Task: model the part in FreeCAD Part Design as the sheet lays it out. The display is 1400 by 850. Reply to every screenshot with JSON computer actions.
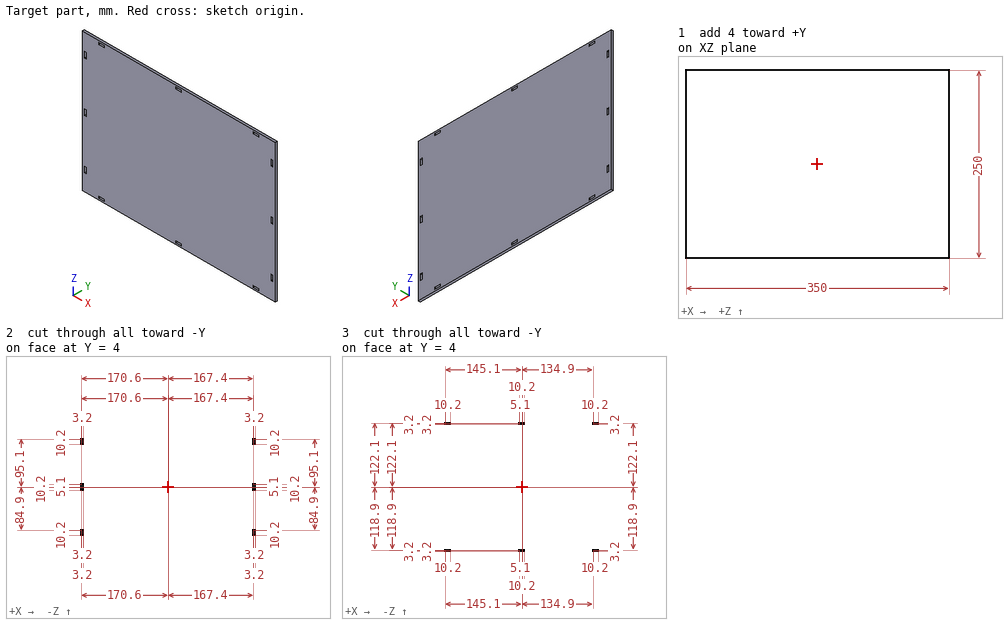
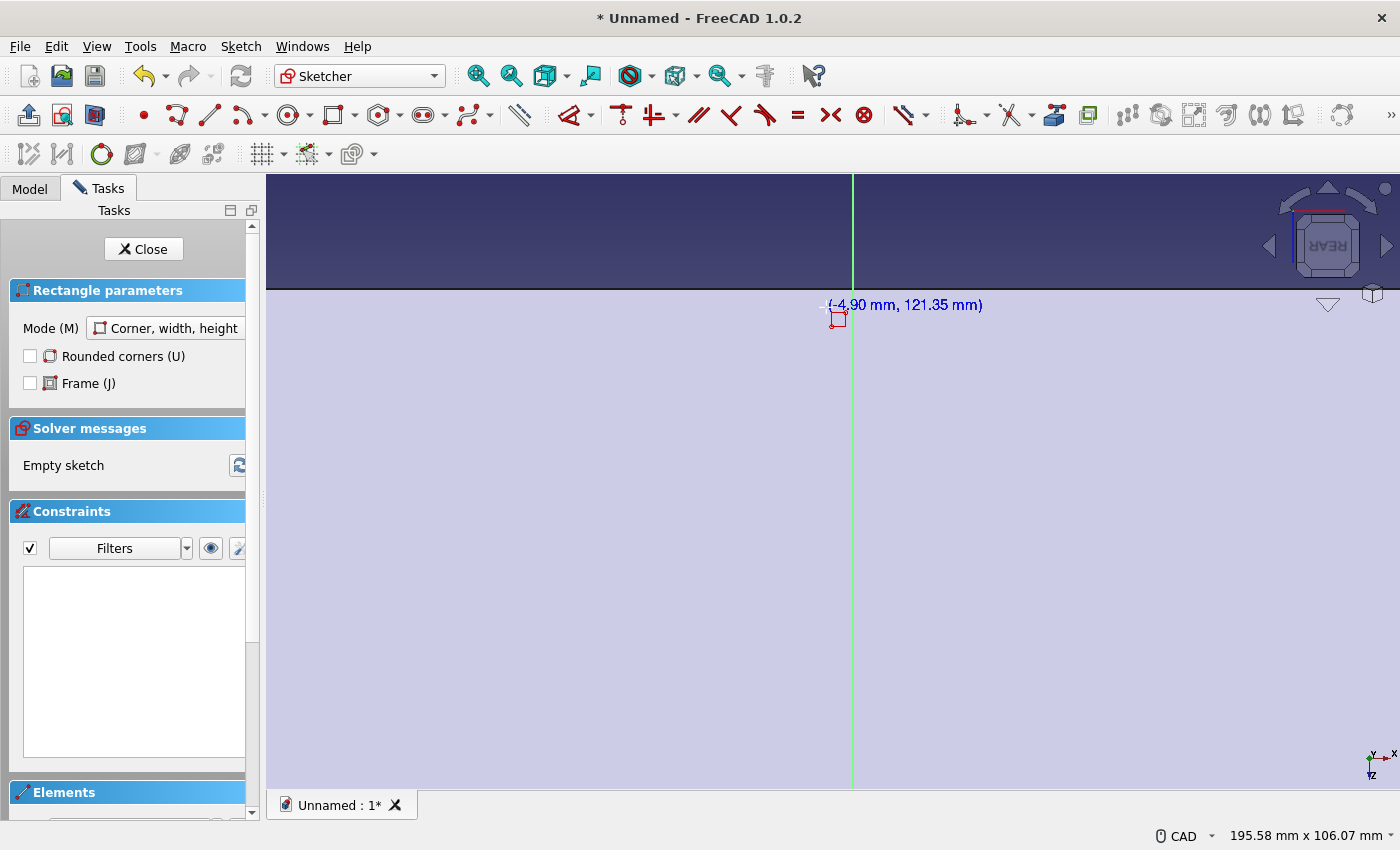
{"action": "left_click", "coordinate": [823, 306]}
{"action": "left_click", "coordinate": [882, 325]}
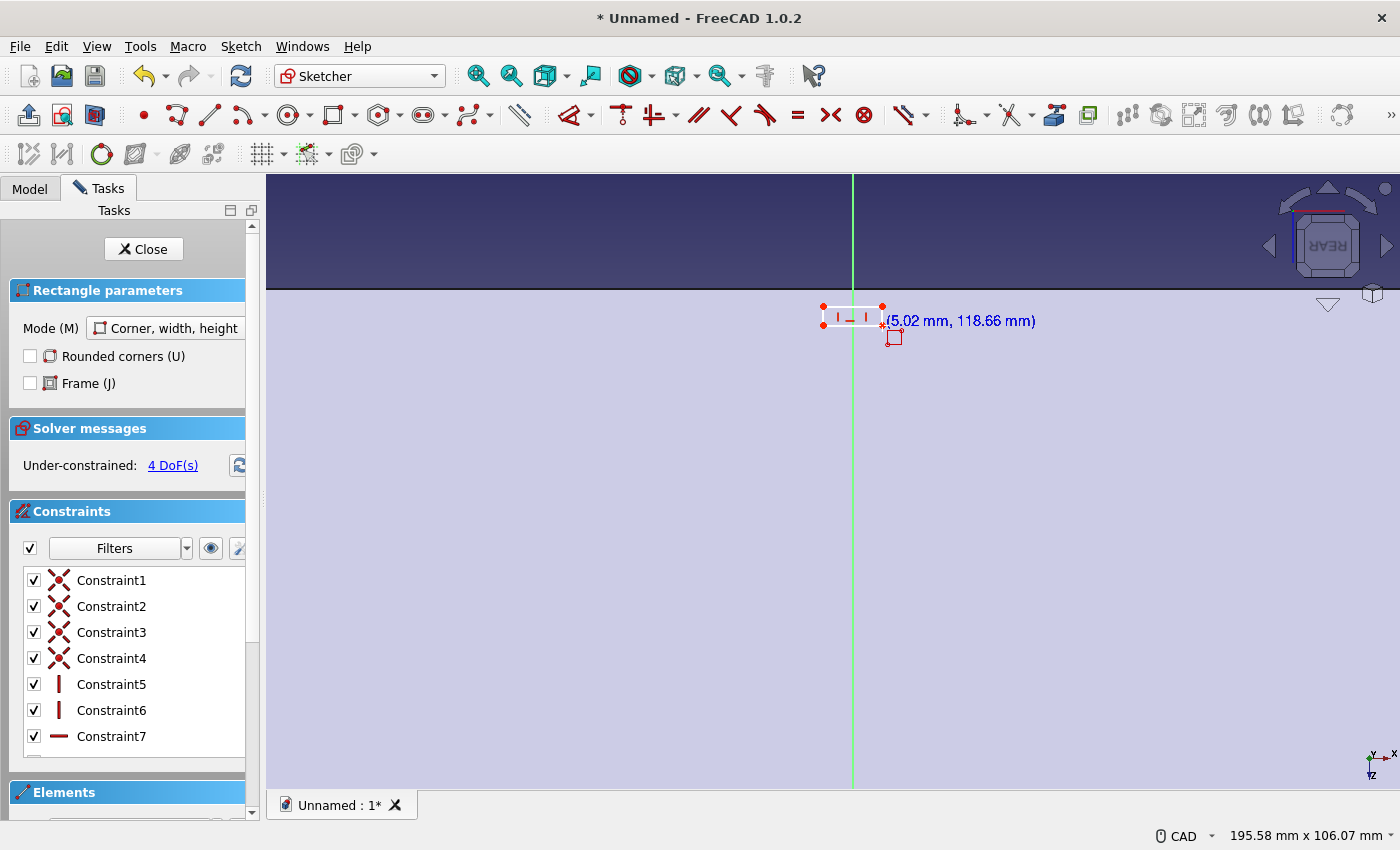
{"action": "scroll", "coordinate": [726, 252], "scroll_direction": "down", "scroll_amount": 6}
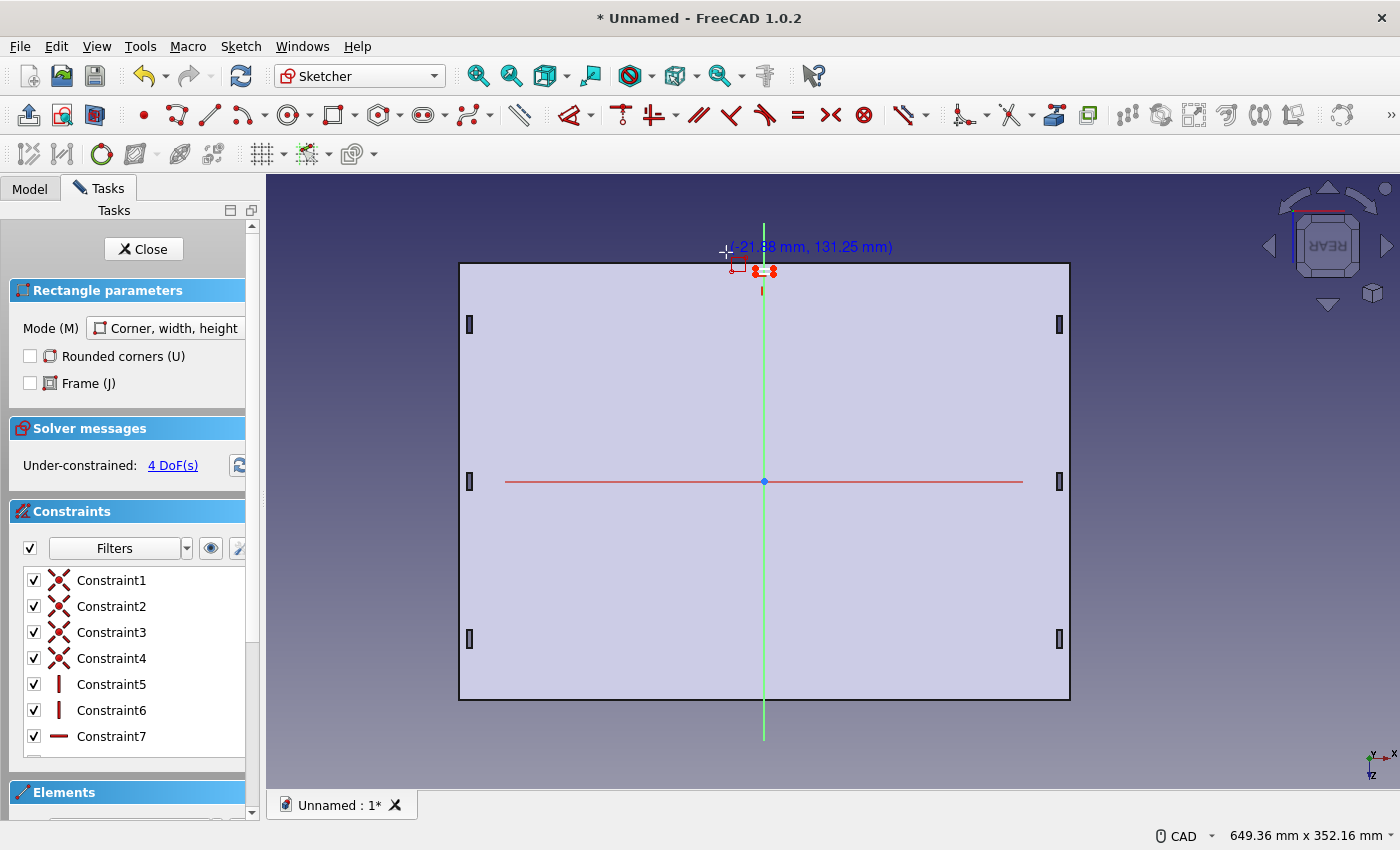
{"action": "scroll", "coordinate": [1000, 268], "scroll_direction": "up", "scroll_amount": 6}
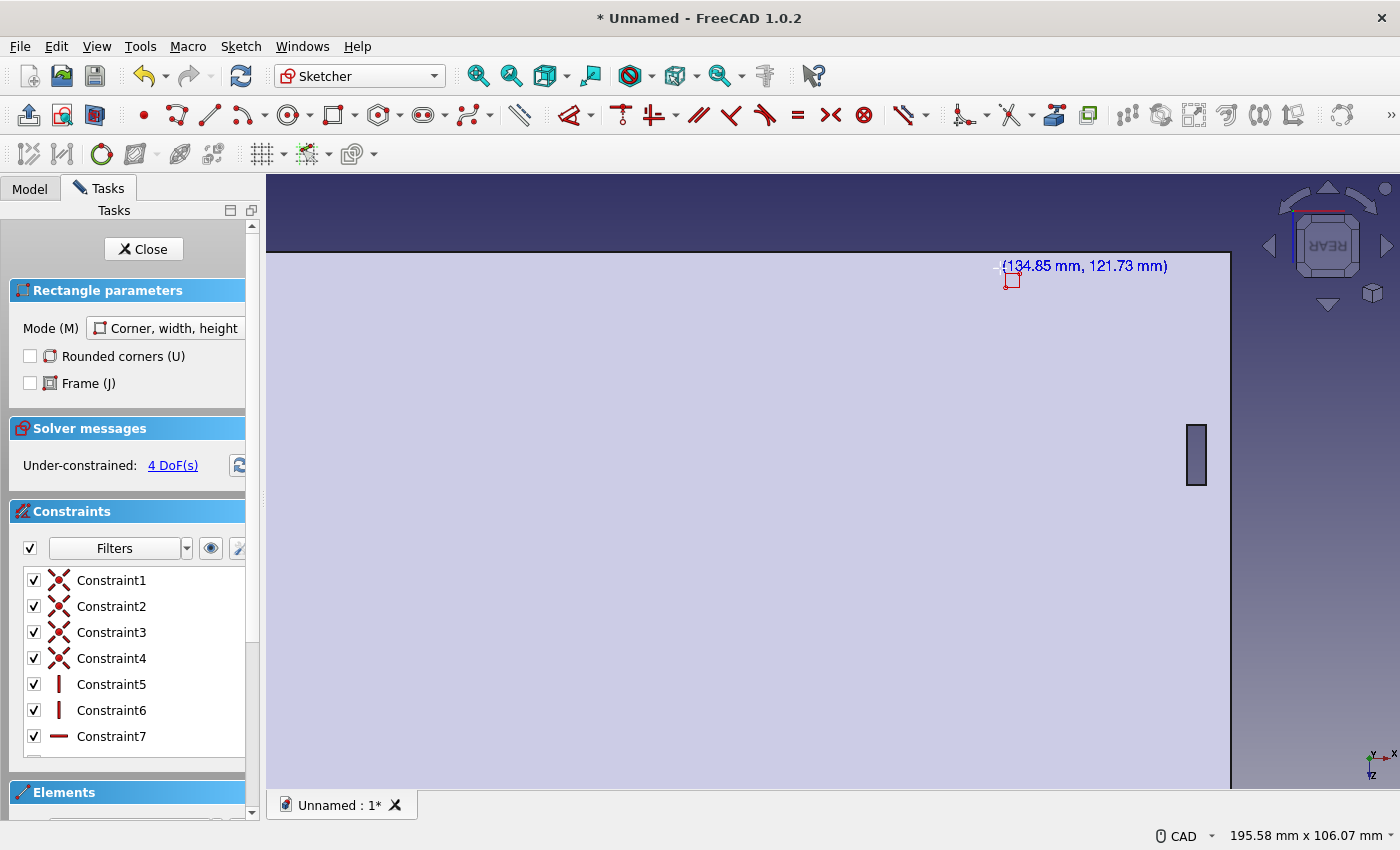
{"action": "scroll", "coordinate": [1001, 268], "scroll_direction": "down", "scroll_amount": 6}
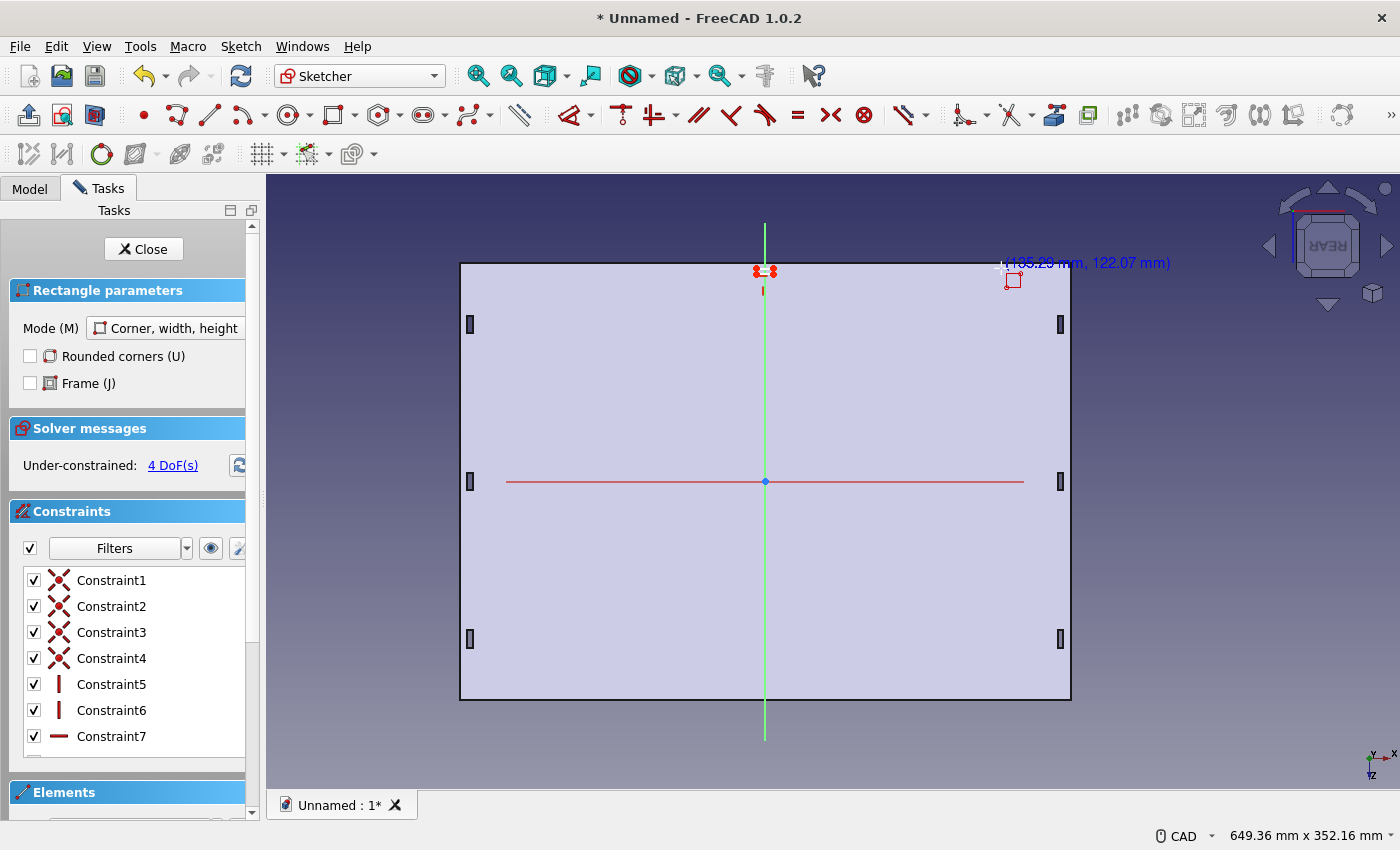
{"action": "left_click", "coordinate": [1001, 268]}
{"action": "left_click", "coordinate": [1019, 274]}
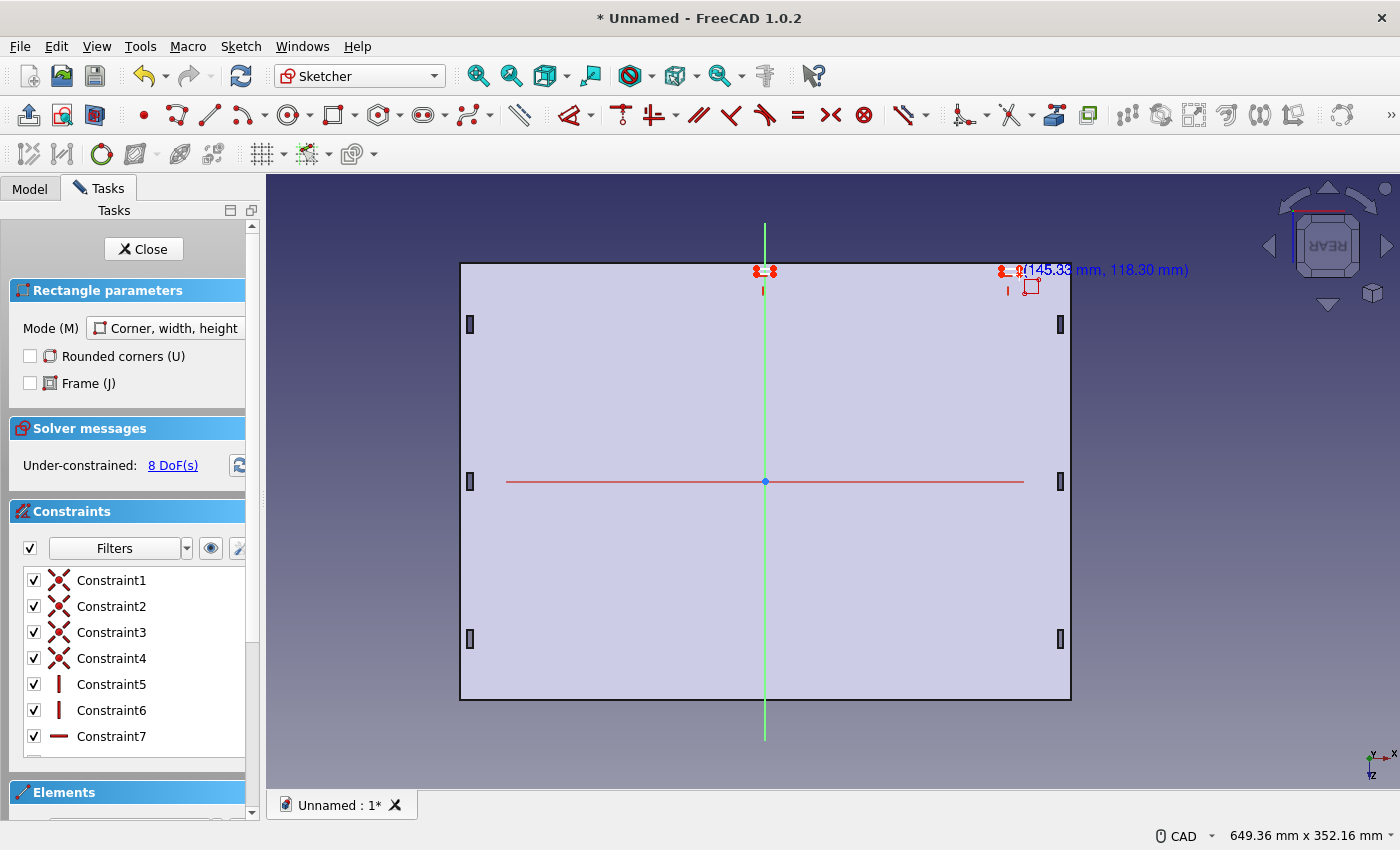
{"action": "scroll", "coordinate": [512, 268], "scroll_direction": "up", "scroll_amount": 6}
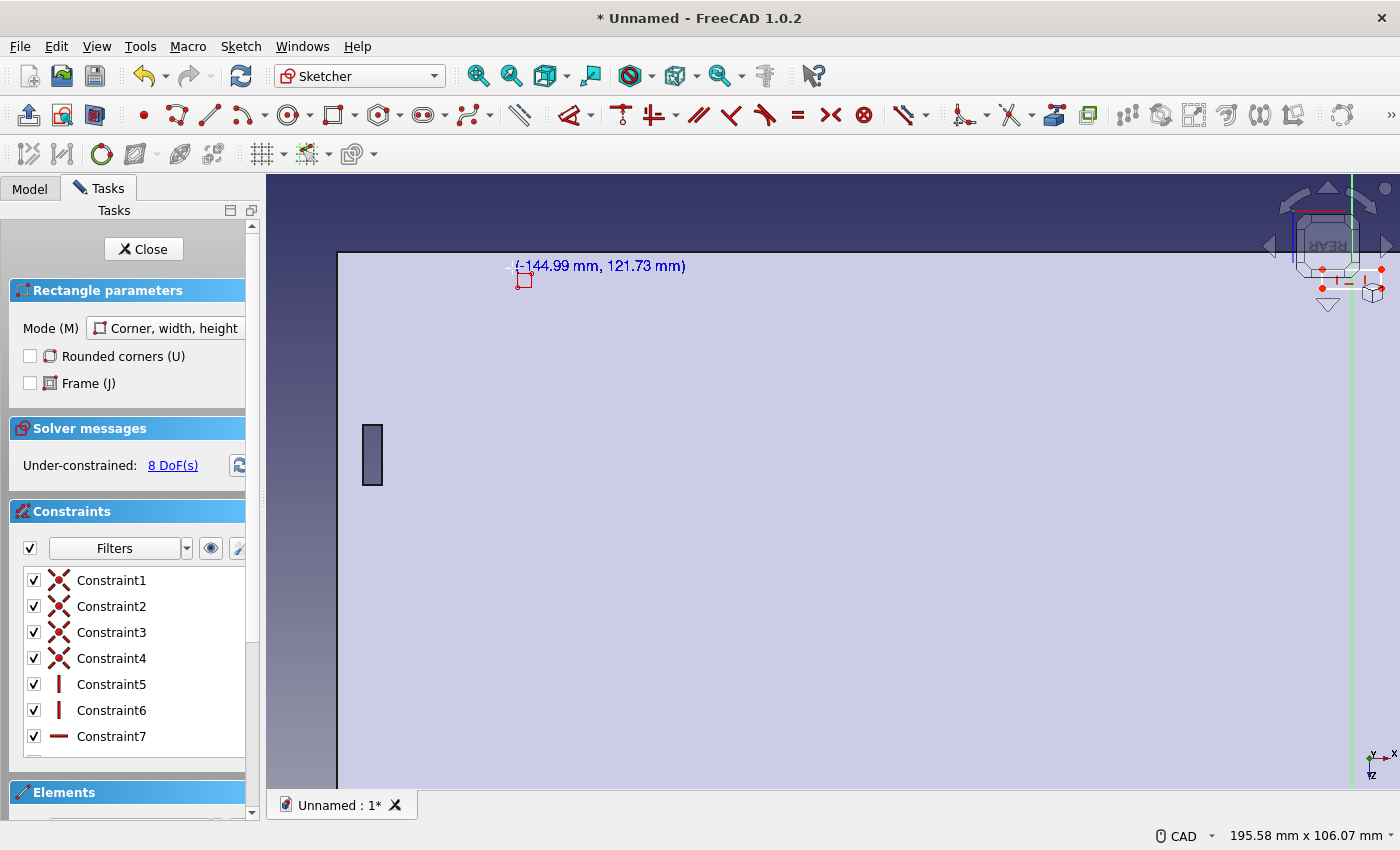
{"action": "scroll", "coordinate": [511, 268], "scroll_direction": "down", "scroll_amount": 6}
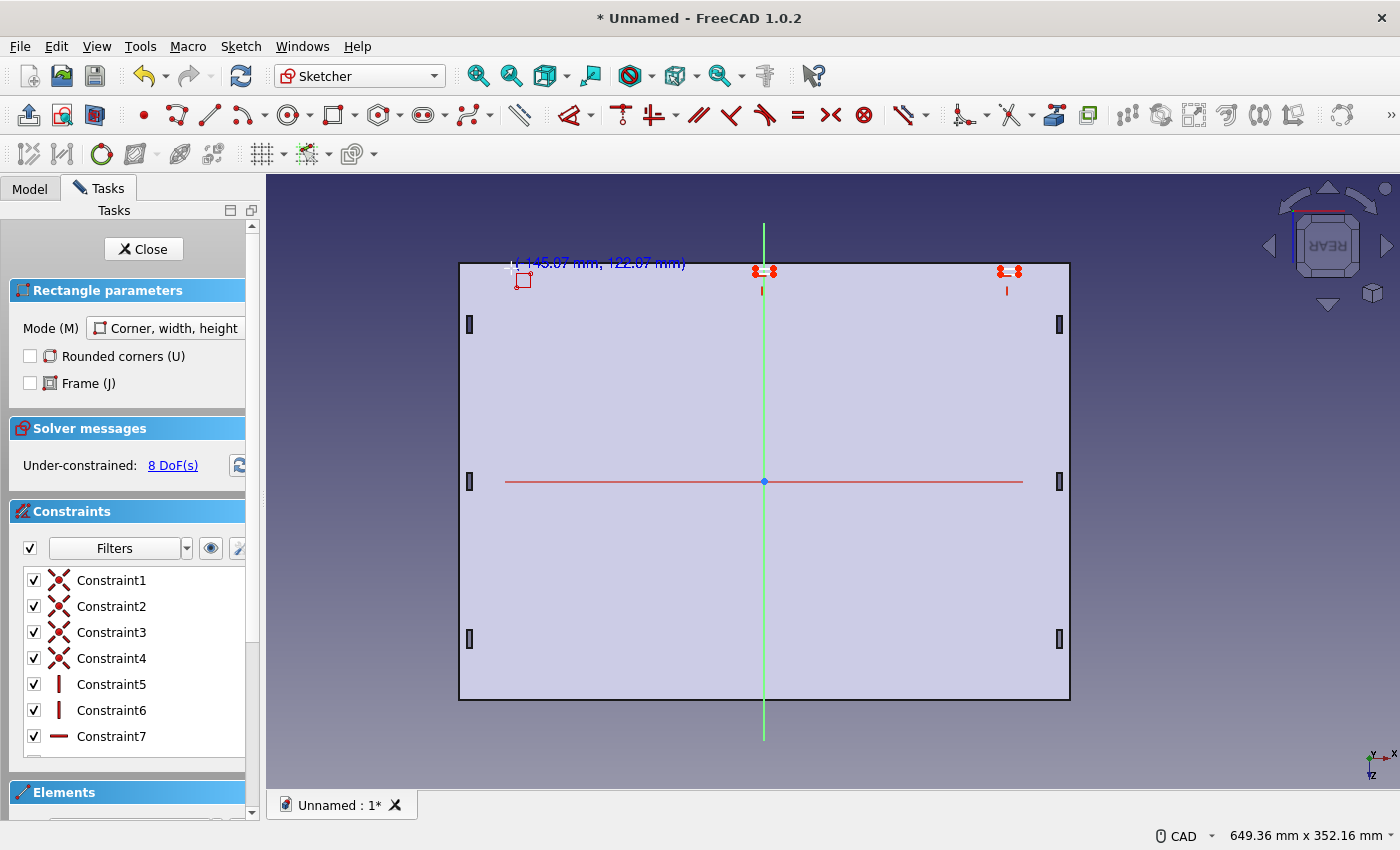
{"action": "left_click", "coordinate": [511, 268]}
{"action": "left_click", "coordinate": [529, 274]}